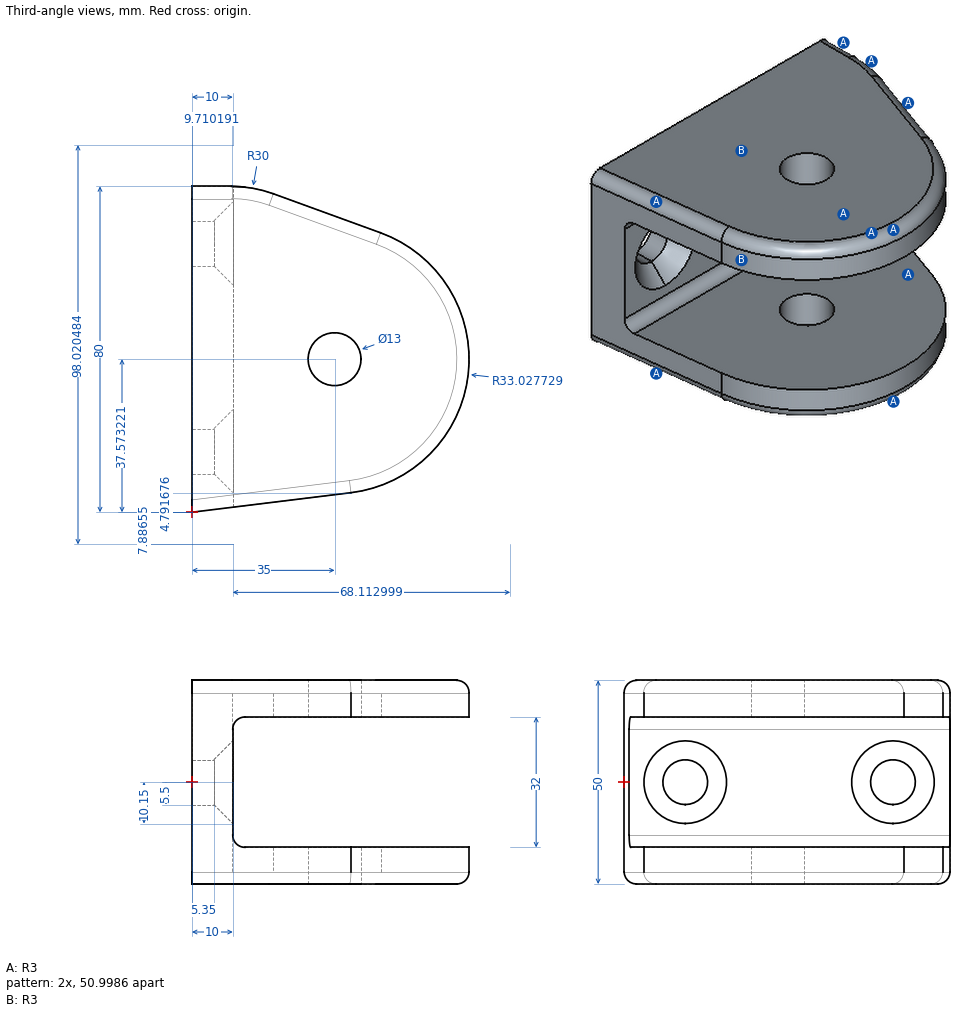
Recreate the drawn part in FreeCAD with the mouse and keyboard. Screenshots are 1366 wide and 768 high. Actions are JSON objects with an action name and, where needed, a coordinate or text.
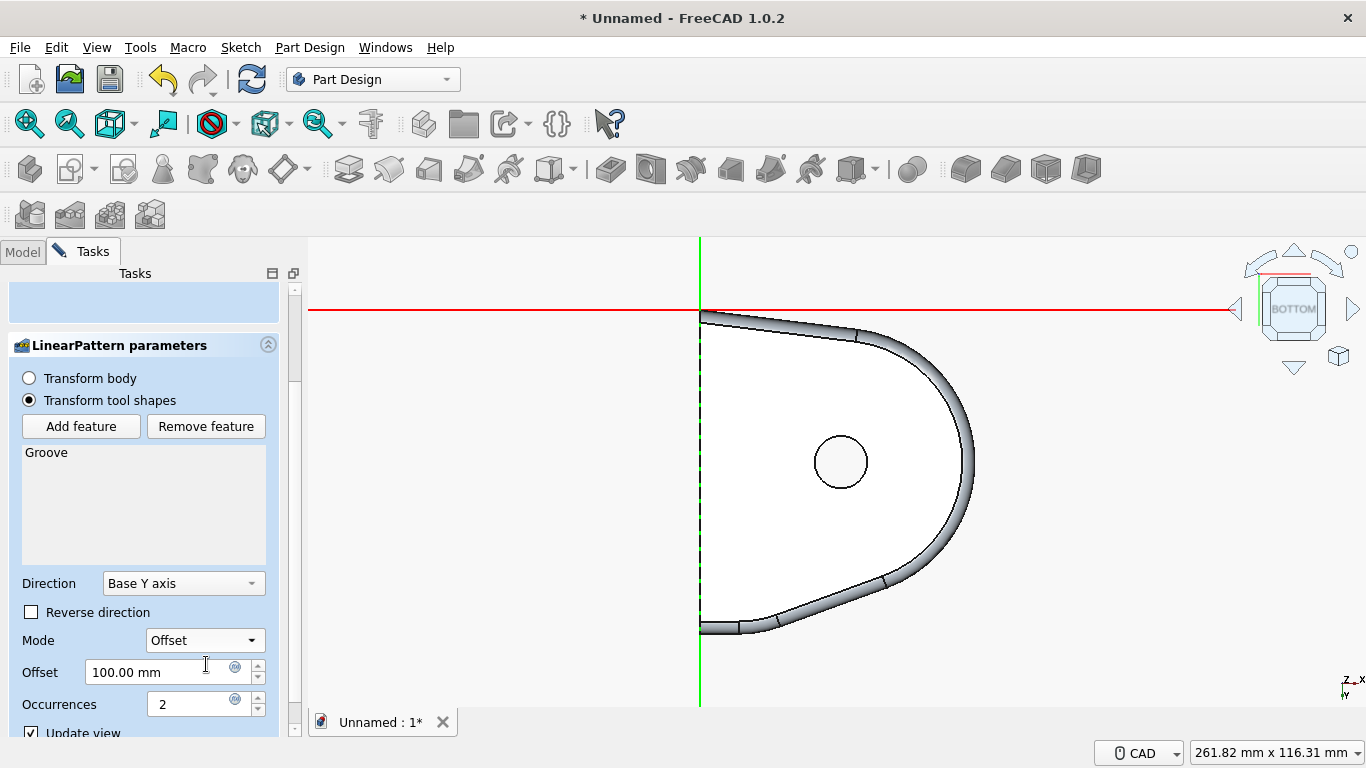
{"action": "triple_click", "coordinate": [168, 672]}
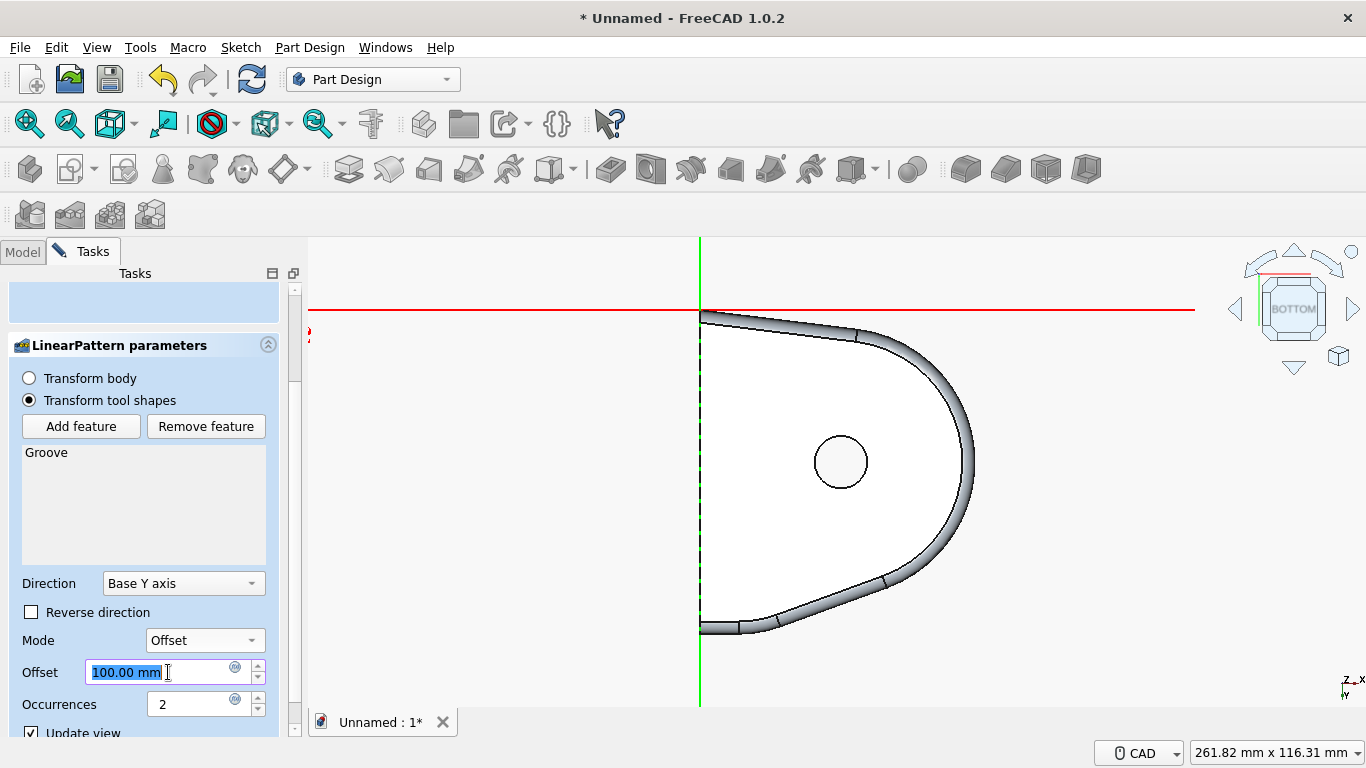
{"action": "type", "text": "50.9986"}
{"action": "key", "text": "Tab"}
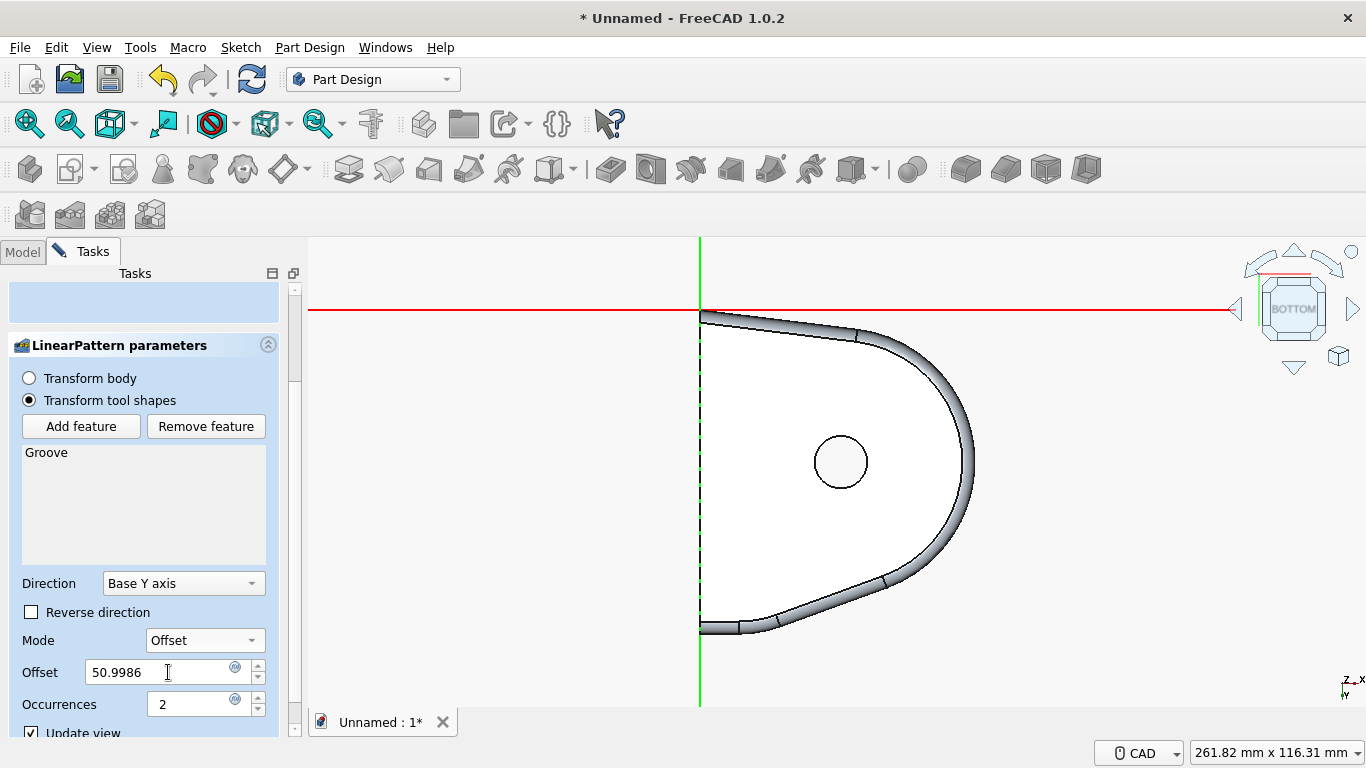
{"action": "triple_click", "coordinate": [198, 704]}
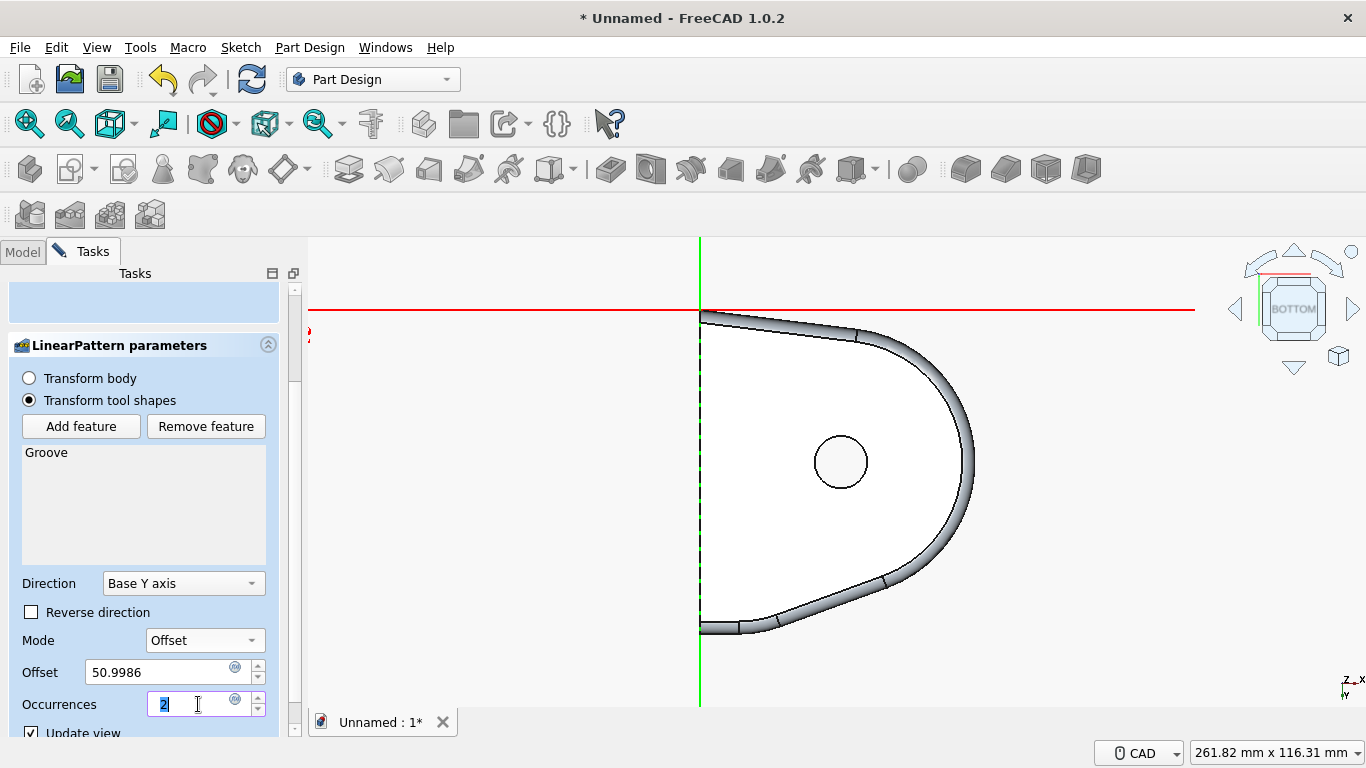
{"action": "type", "text": "2"}
{"action": "key", "text": "Tab"}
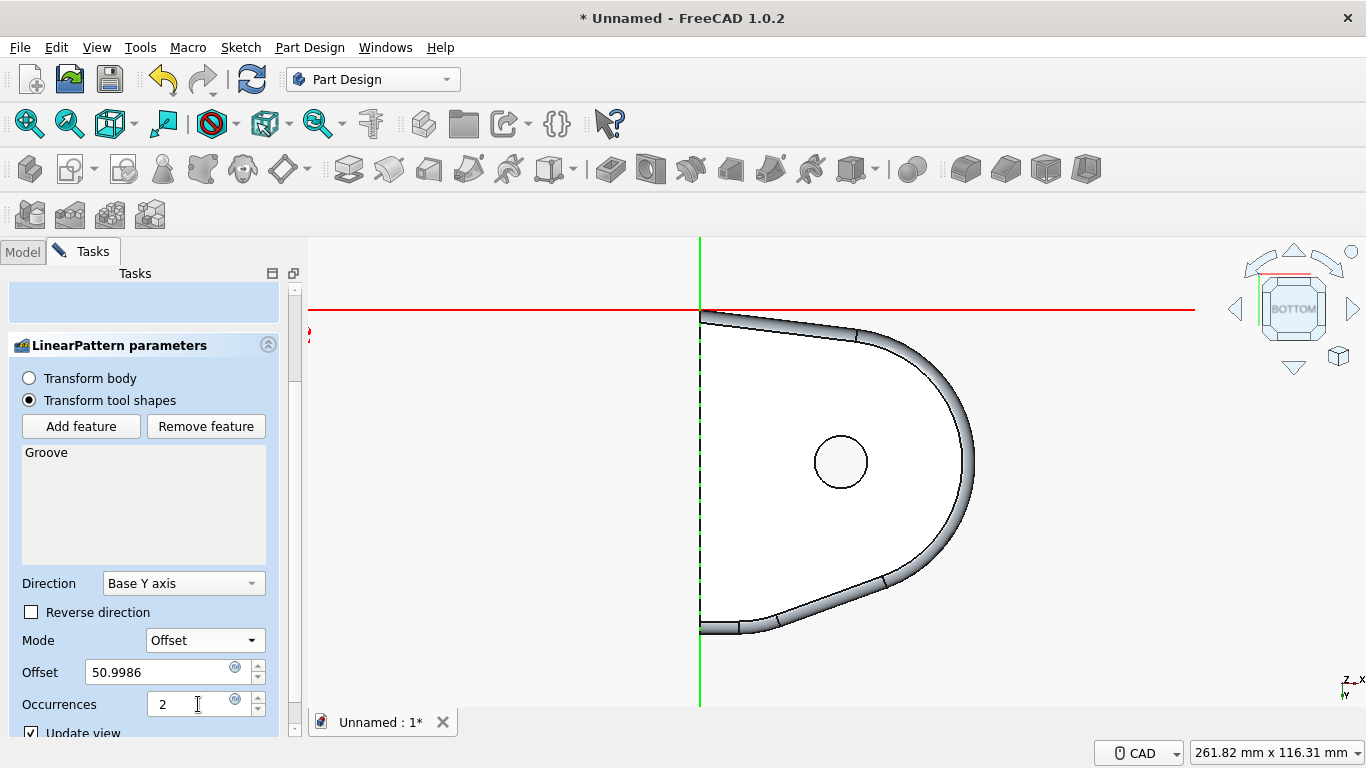
{"action": "left_click", "coordinate": [30, 612]}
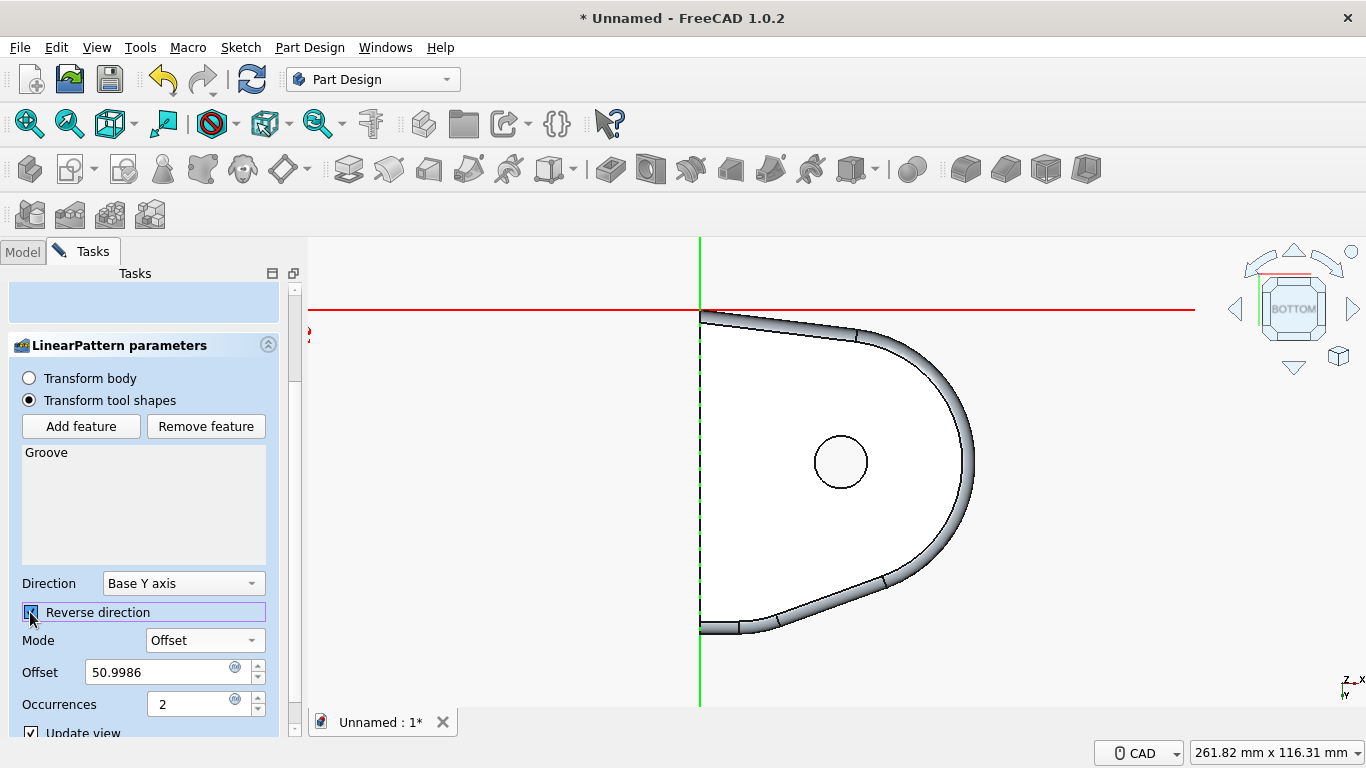
{"action": "scroll", "coordinate": [295, 510], "scroll_direction": "up", "scroll_amount": 3}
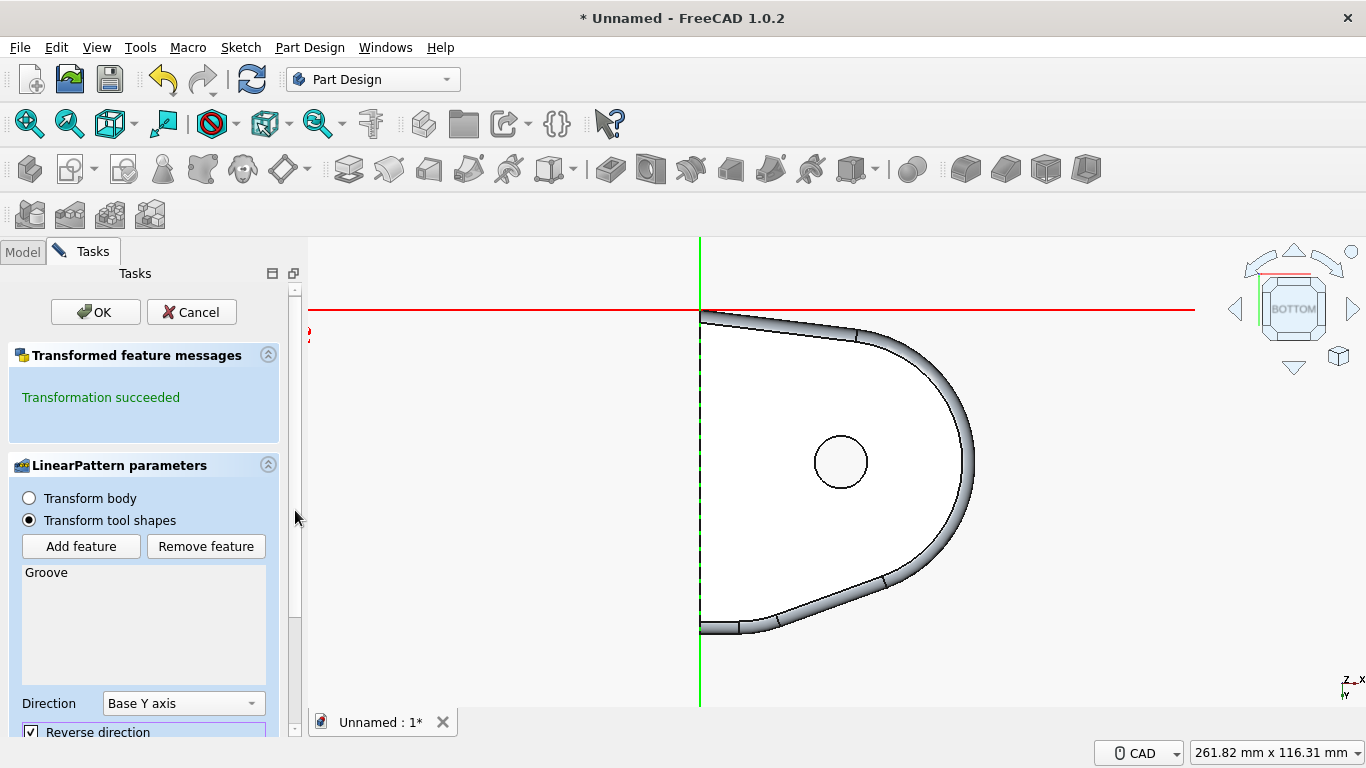
{"action": "left_click", "coordinate": [96, 312]}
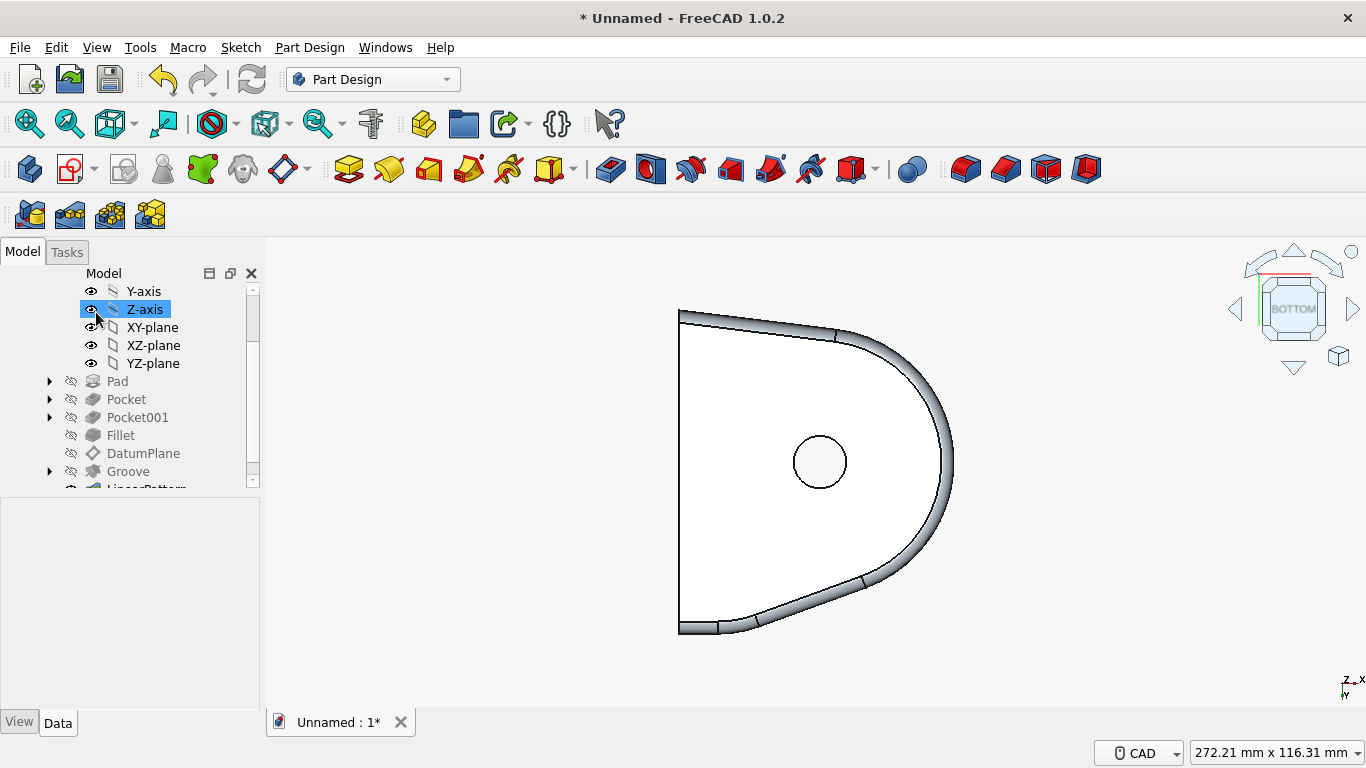
{"action": "key", "text": "0"}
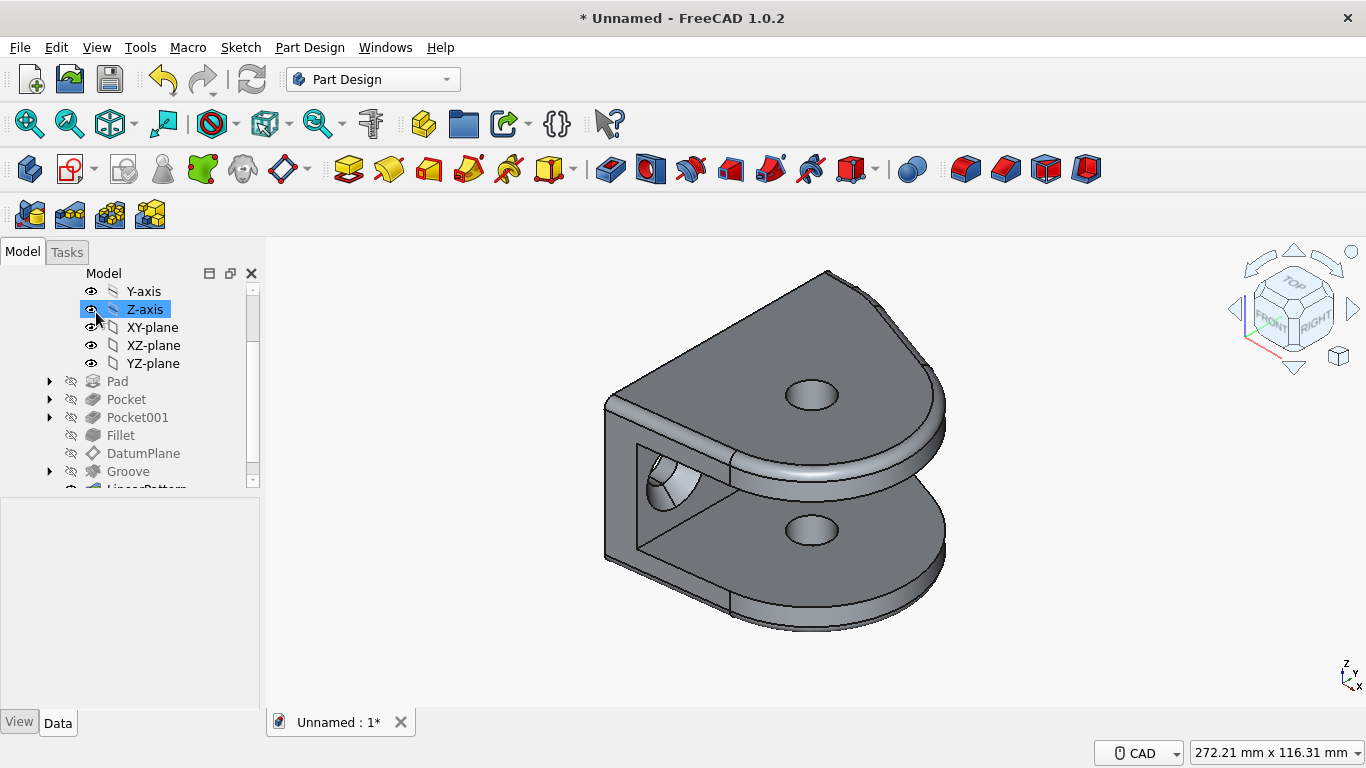
{"action": "key", "text": "2"}